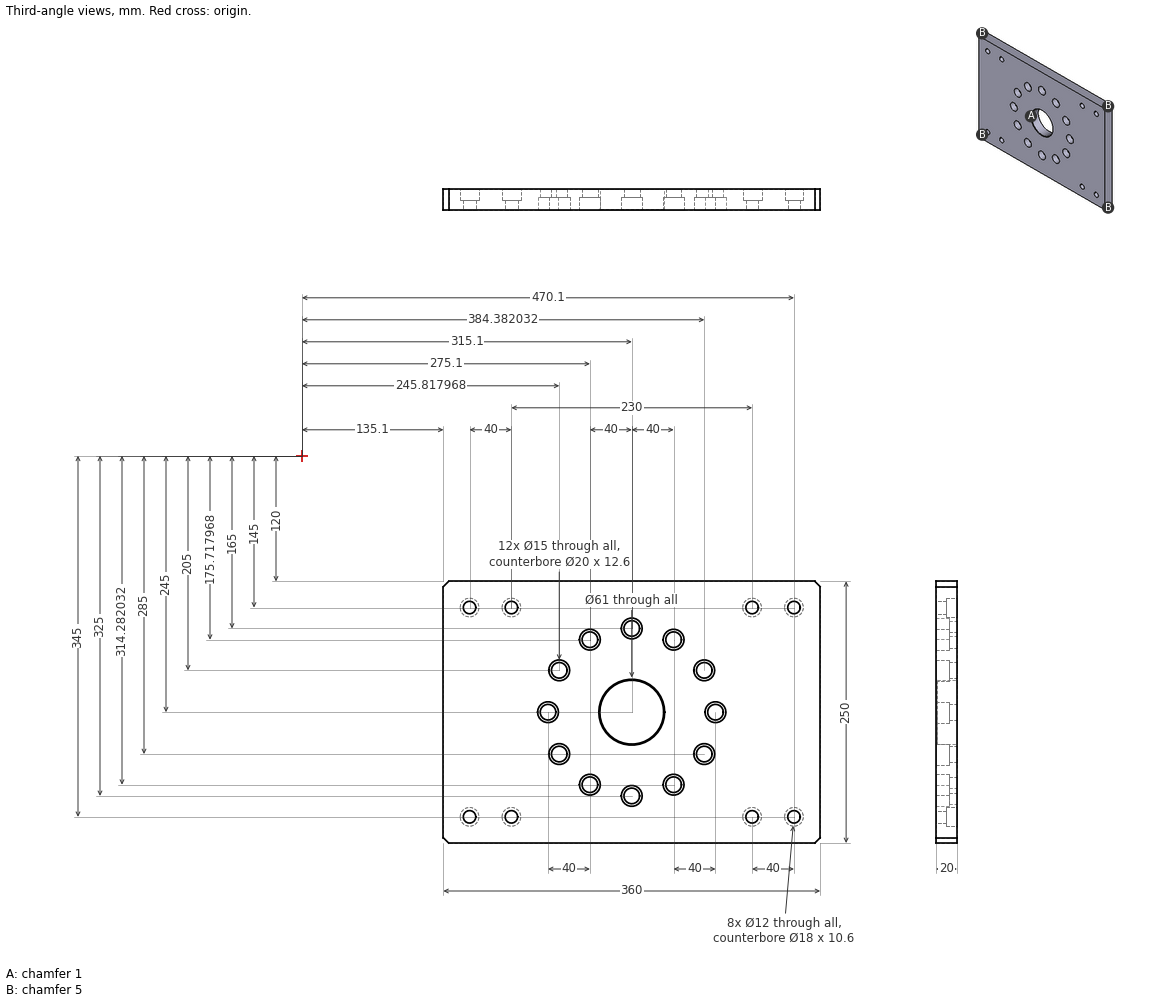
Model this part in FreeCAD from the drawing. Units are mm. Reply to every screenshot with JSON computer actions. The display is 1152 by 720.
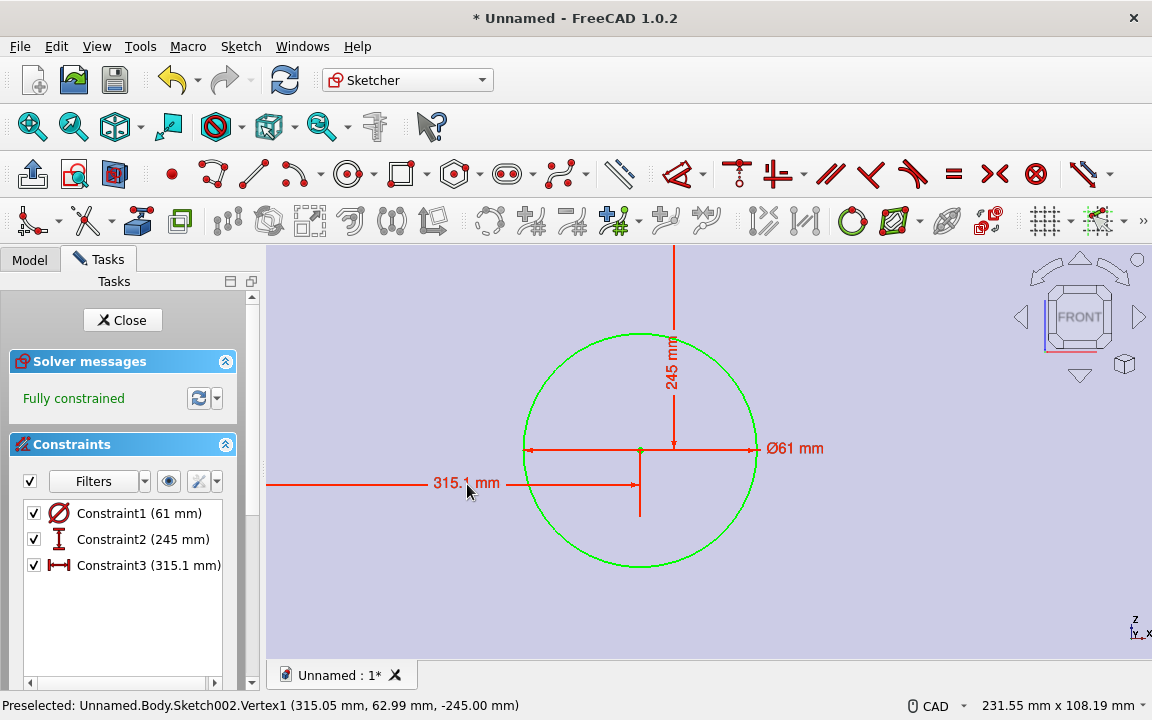
{"action": "left_click", "coordinate": [123, 320]}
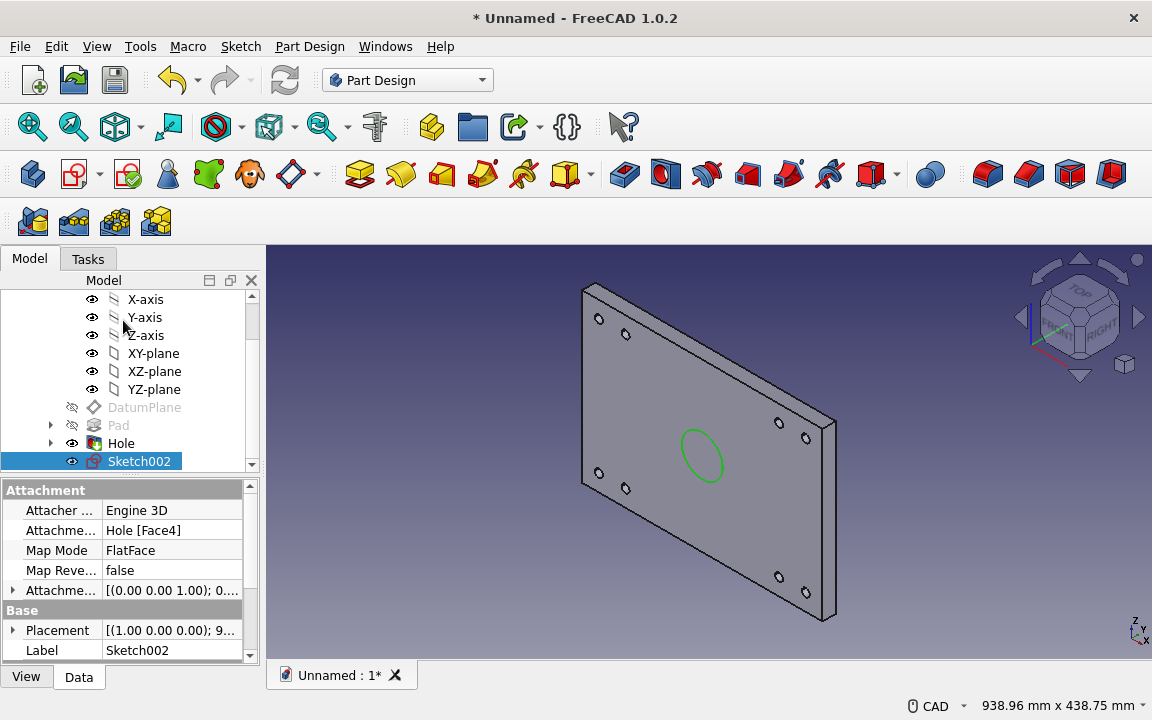
{"action": "left_click", "coordinate": [666, 174]}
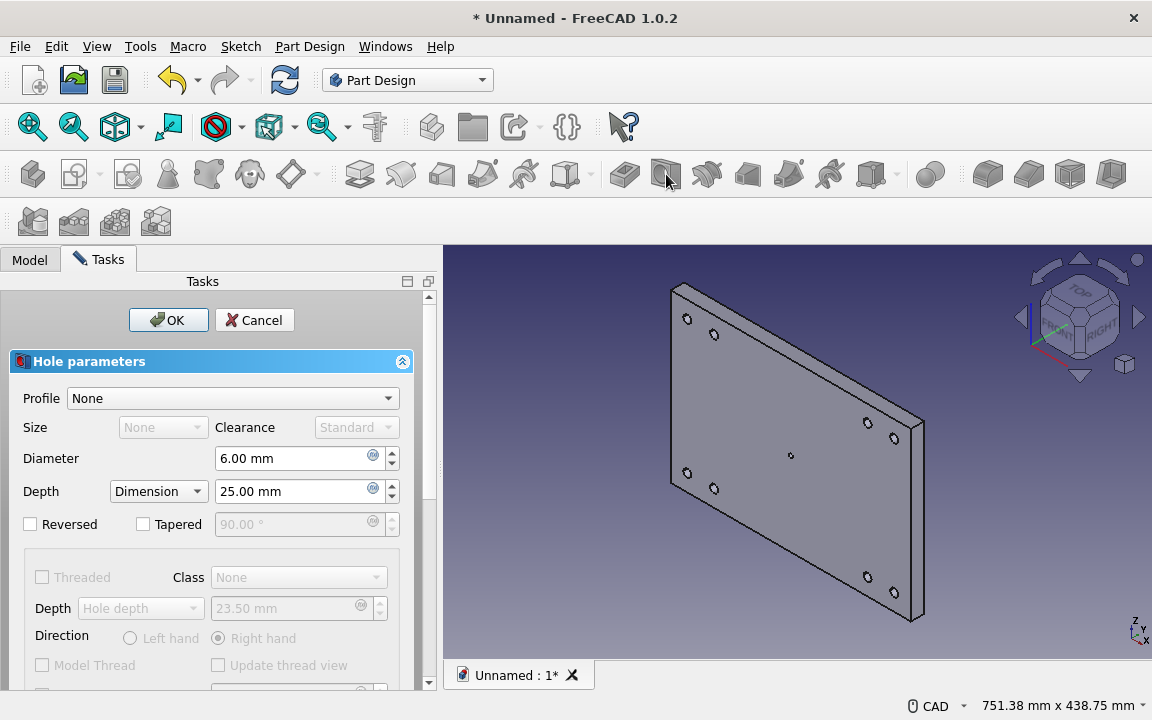
{"action": "triple_click", "coordinate": [300, 458]}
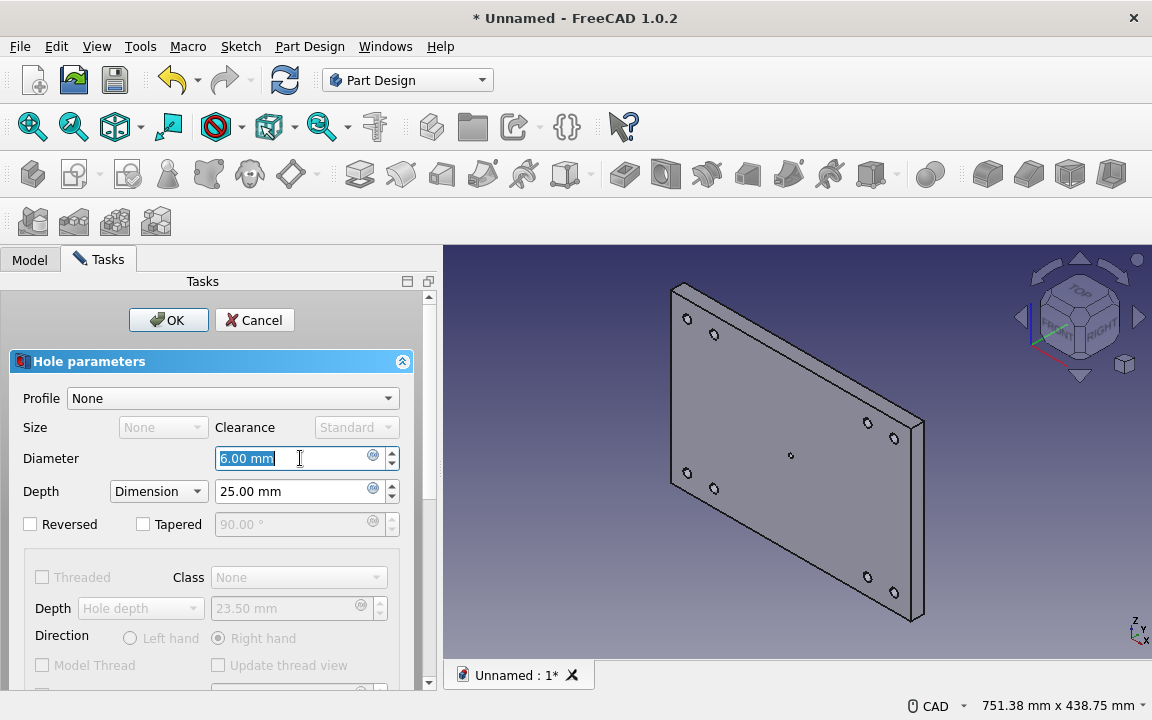
{"action": "type", "text": "61"}
{"action": "key", "text": "Tab"}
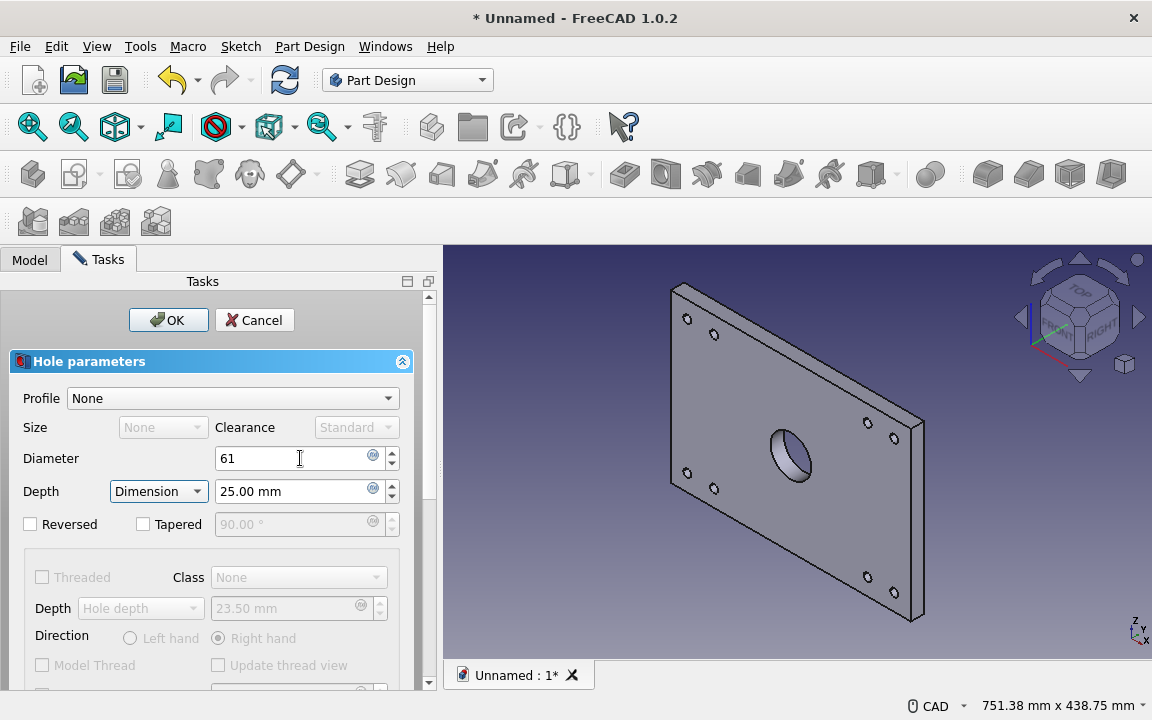
{"action": "left_click", "coordinate": [160, 492]}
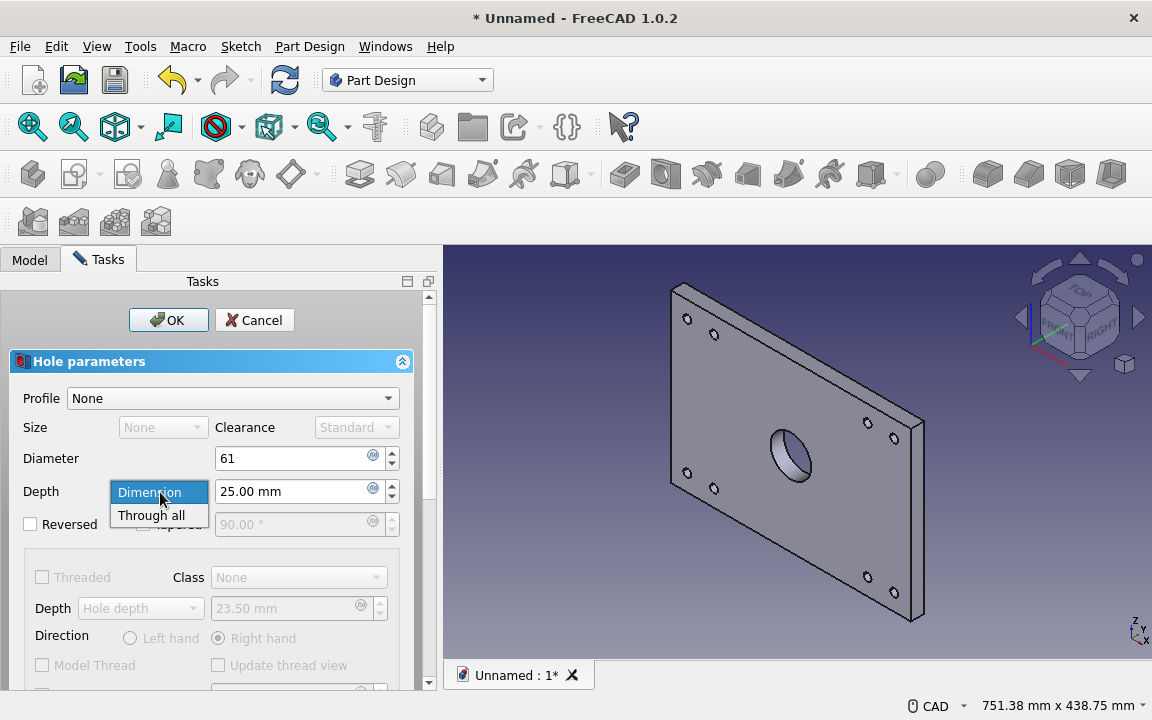
{"action": "left_click", "coordinate": [158, 516]}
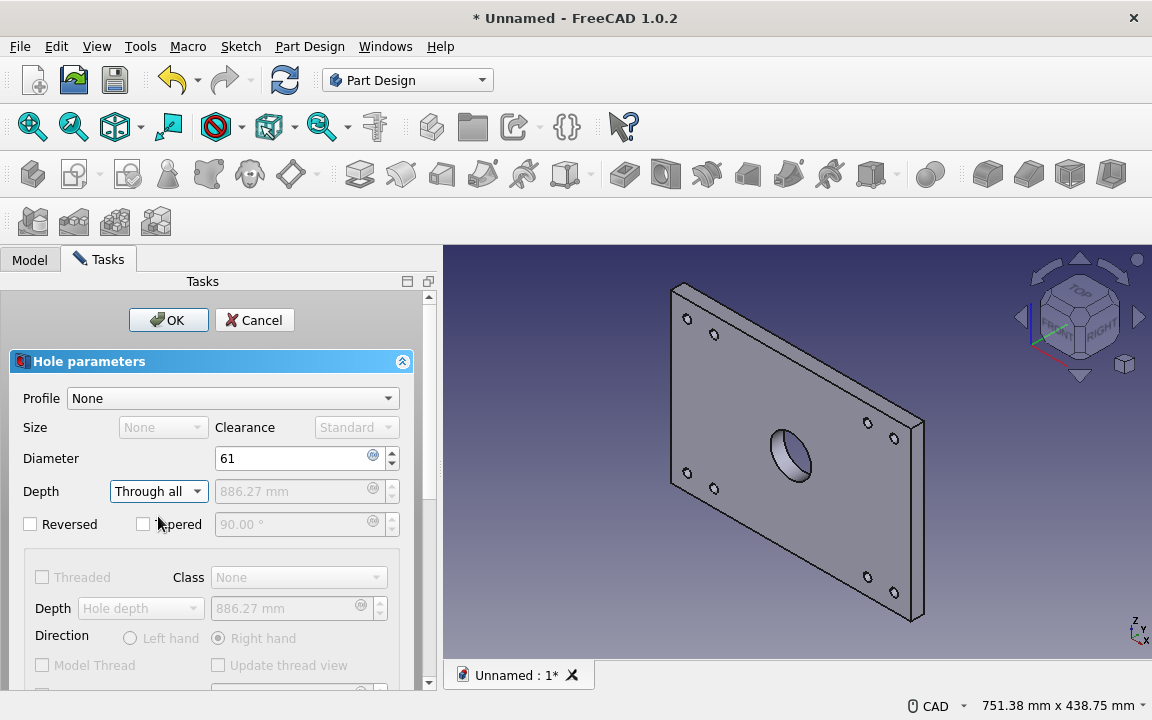
{"action": "left_click", "coordinate": [169, 320]}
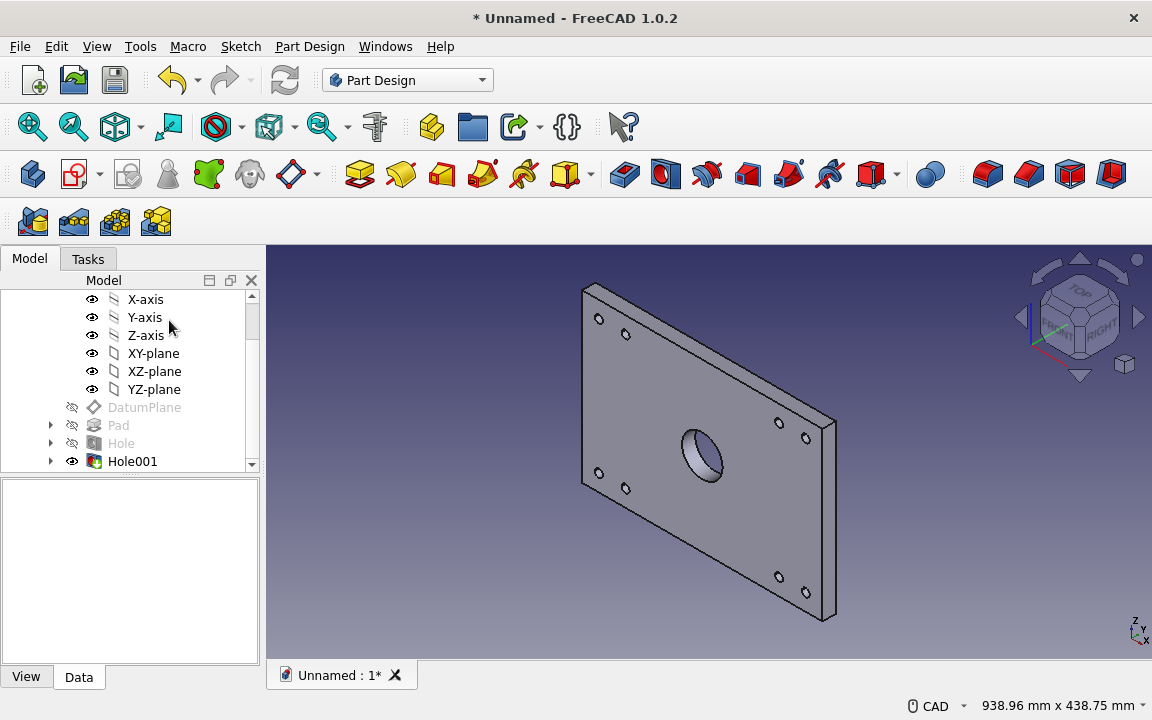
{"action": "left_click", "coordinate": [634, 415]}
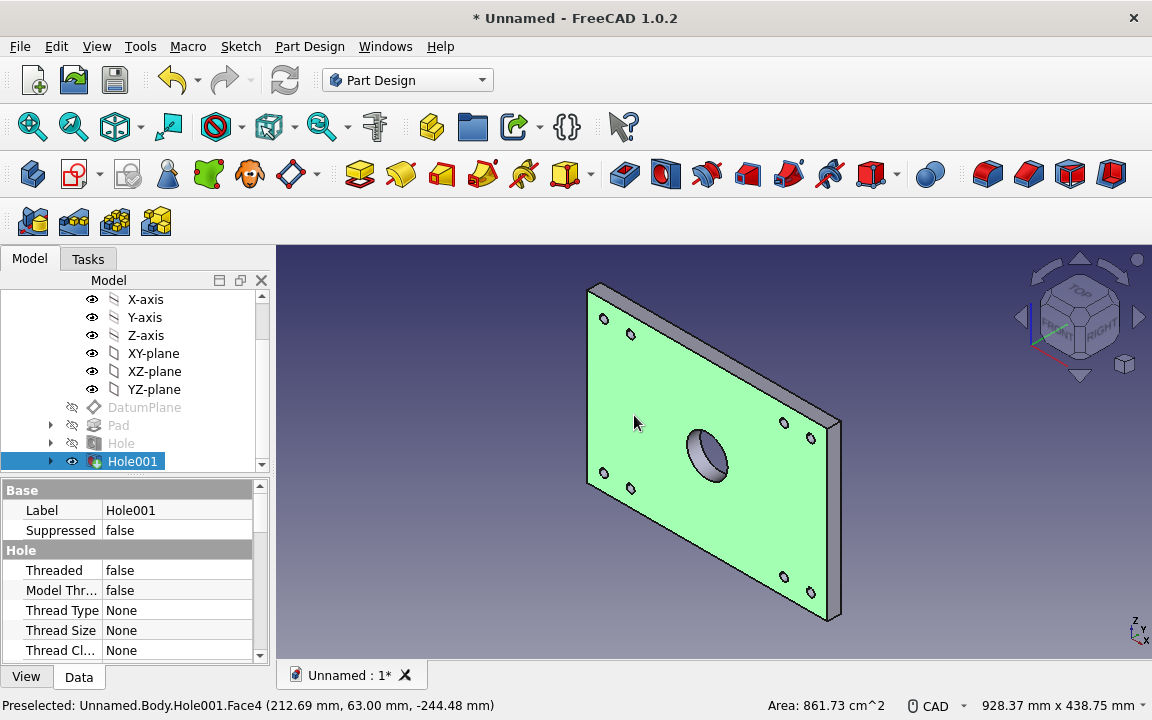
{"action": "left_click", "coordinate": [74, 174]}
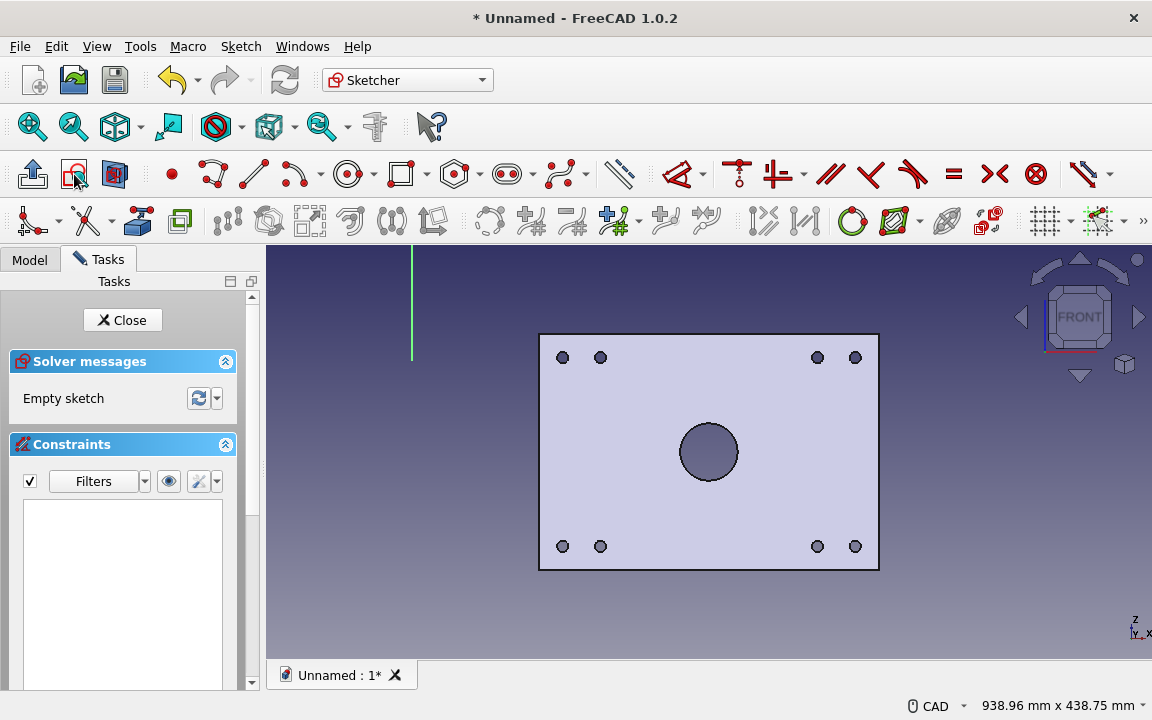
{"action": "scroll", "coordinate": [720, 603], "scroll_direction": "down", "scroll_amount": 2}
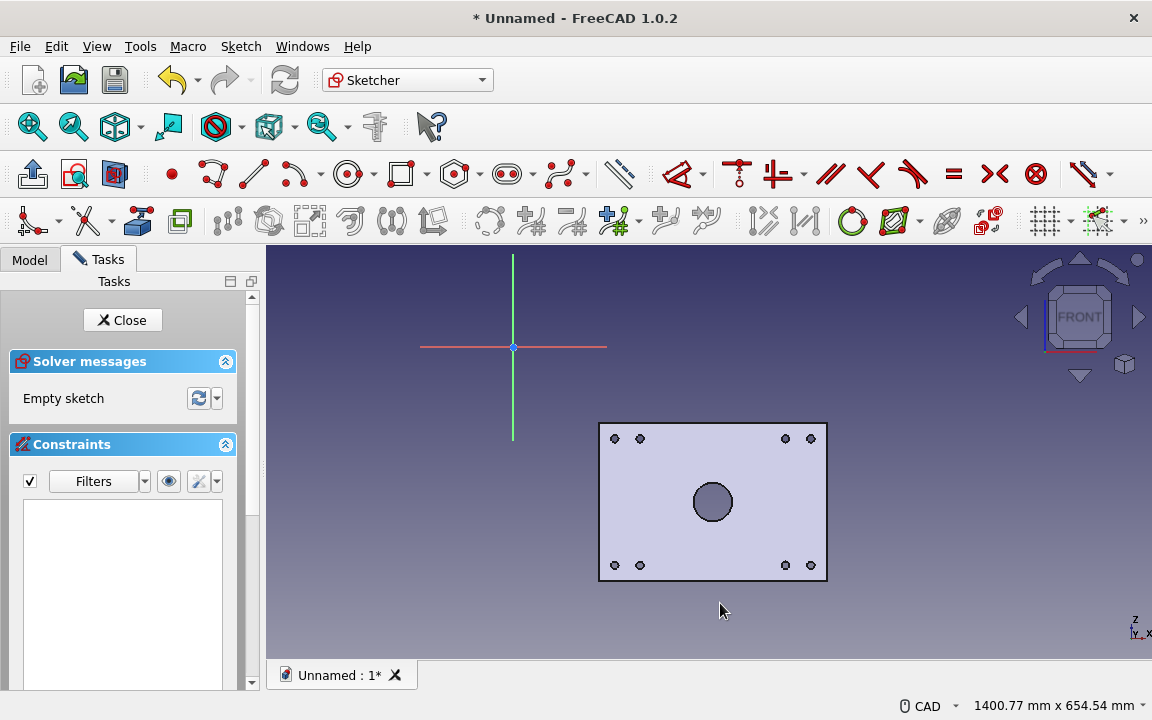
{"action": "left_click", "coordinate": [348, 174]}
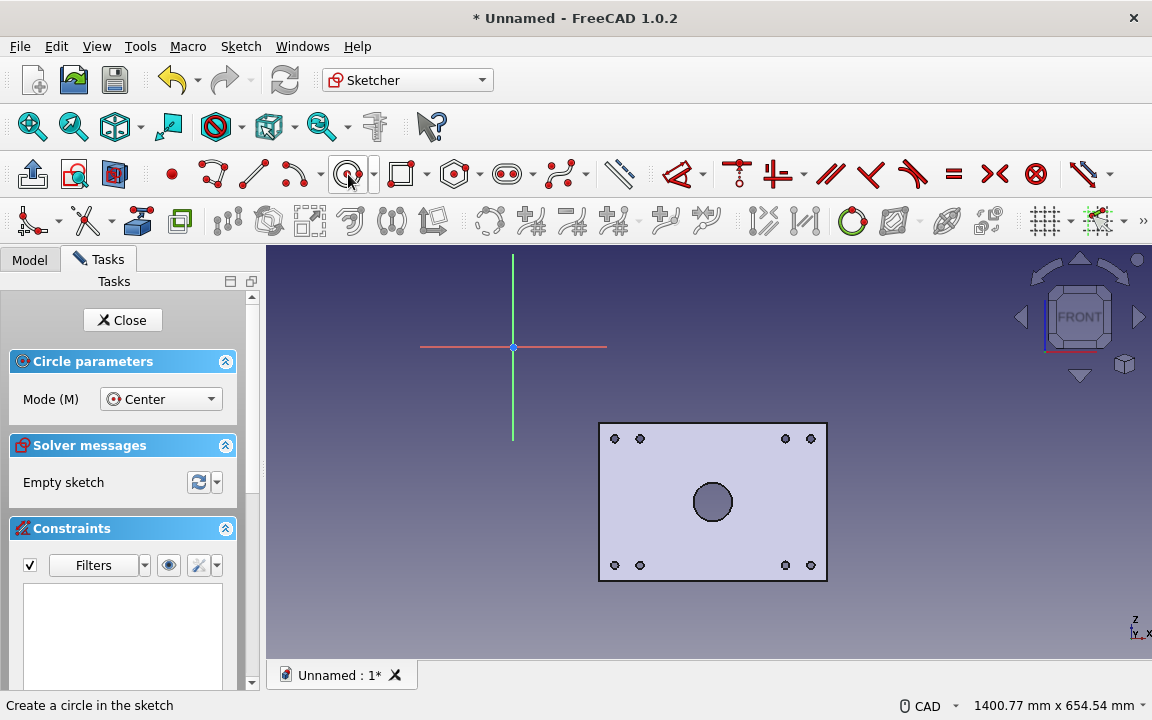
{"action": "scroll", "coordinate": [669, 477], "scroll_direction": "up", "scroll_amount": 8}